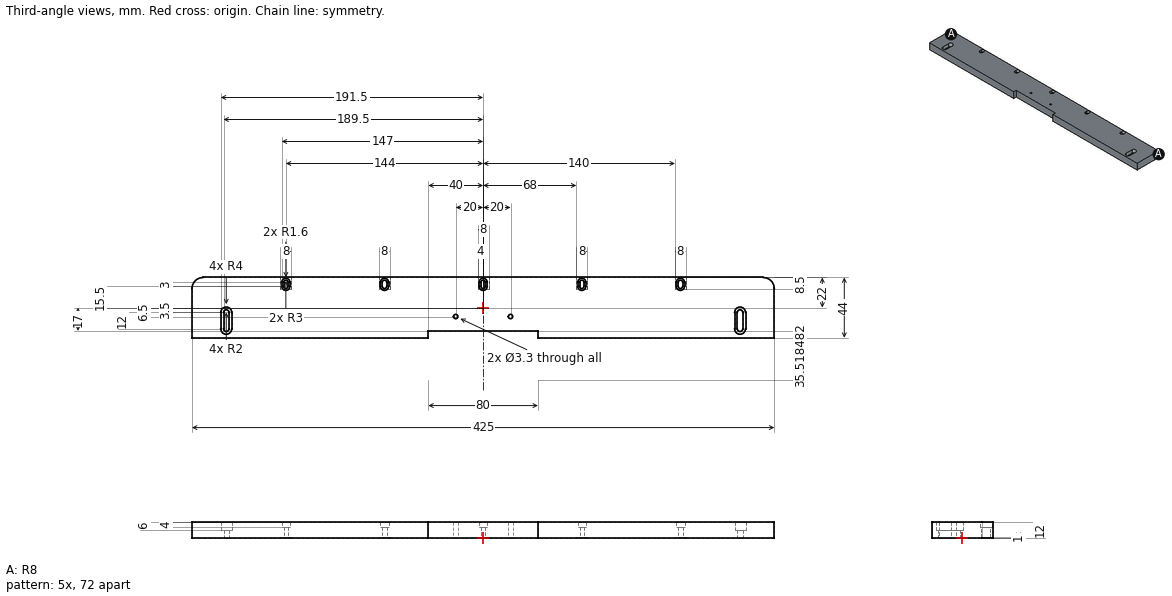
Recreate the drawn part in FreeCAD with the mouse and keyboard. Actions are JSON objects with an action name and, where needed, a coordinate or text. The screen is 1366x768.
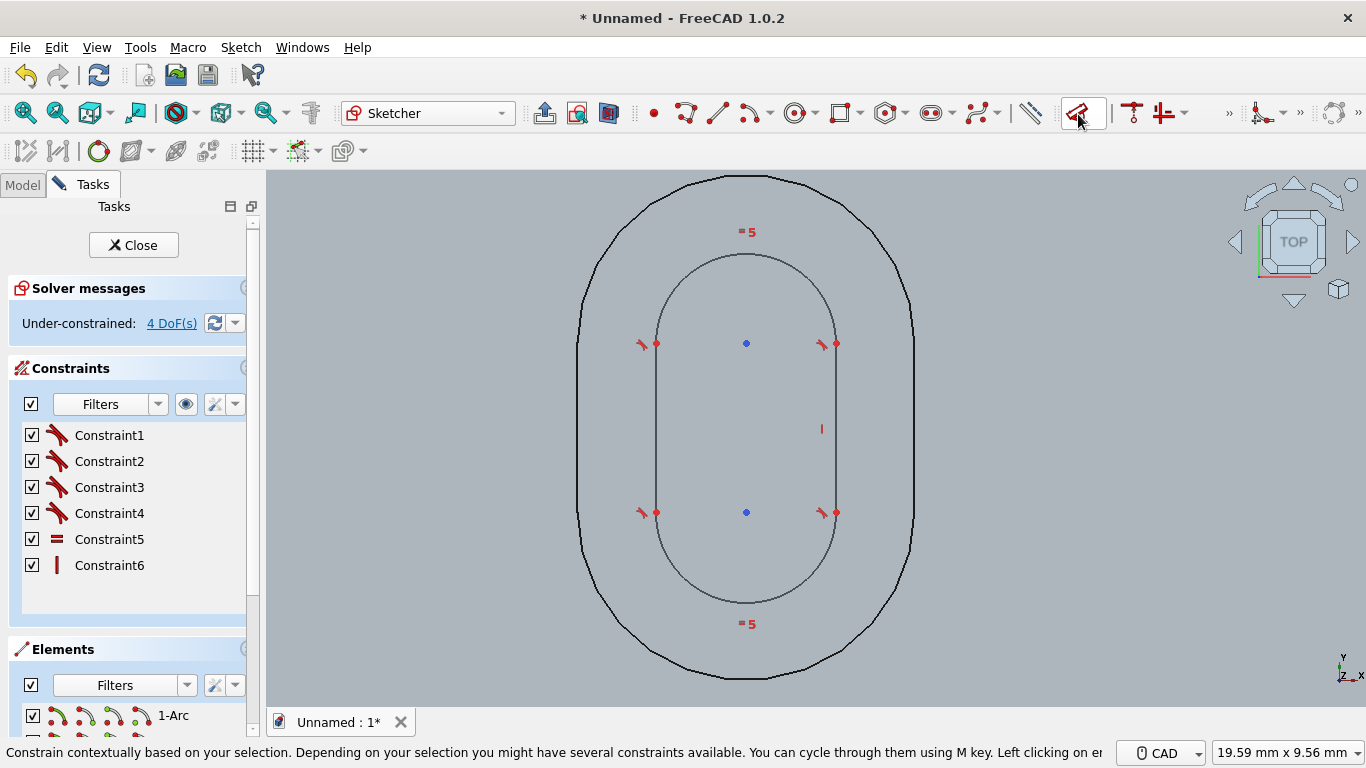
{"action": "left_click", "coordinate": [693, 586]}
{"action": "left_click", "coordinate": [674, 612]}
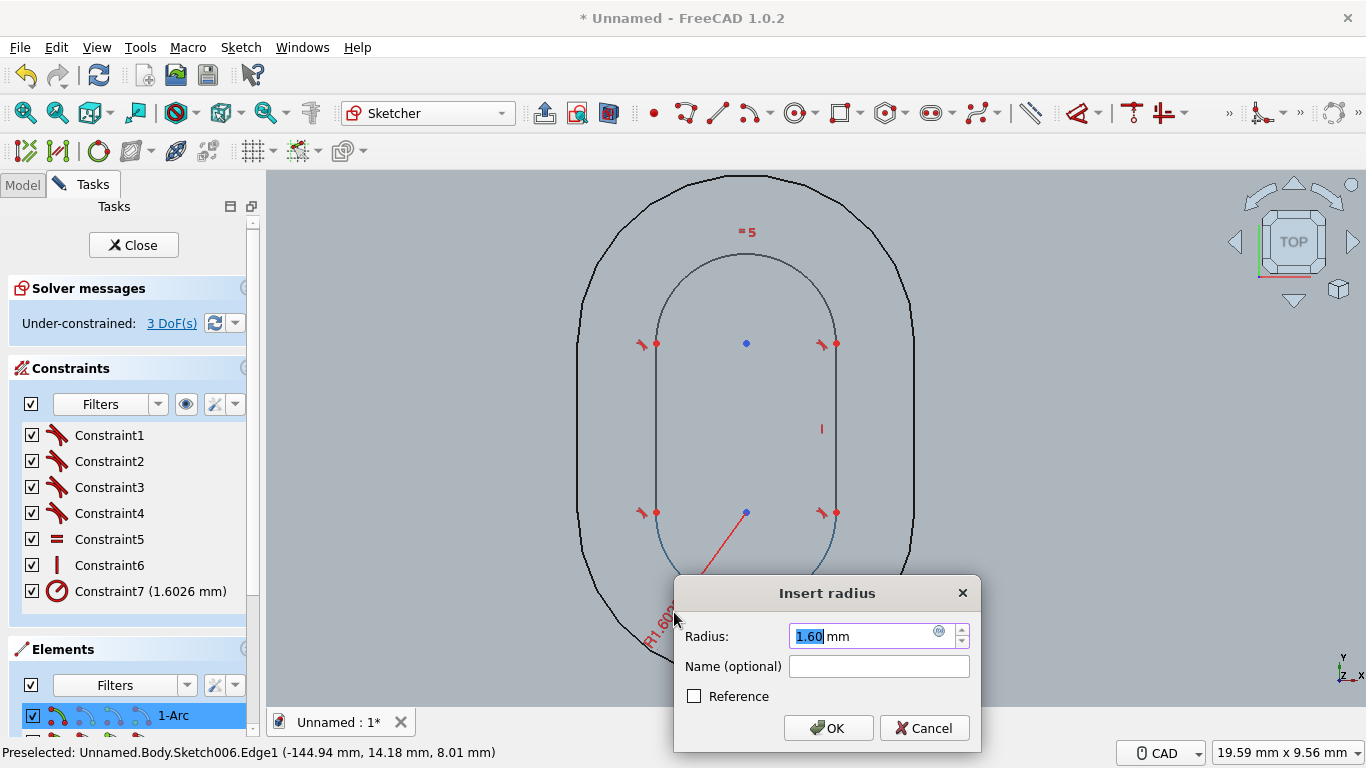
{"action": "type", "text": "1.6"}
{"action": "key", "text": "Return"}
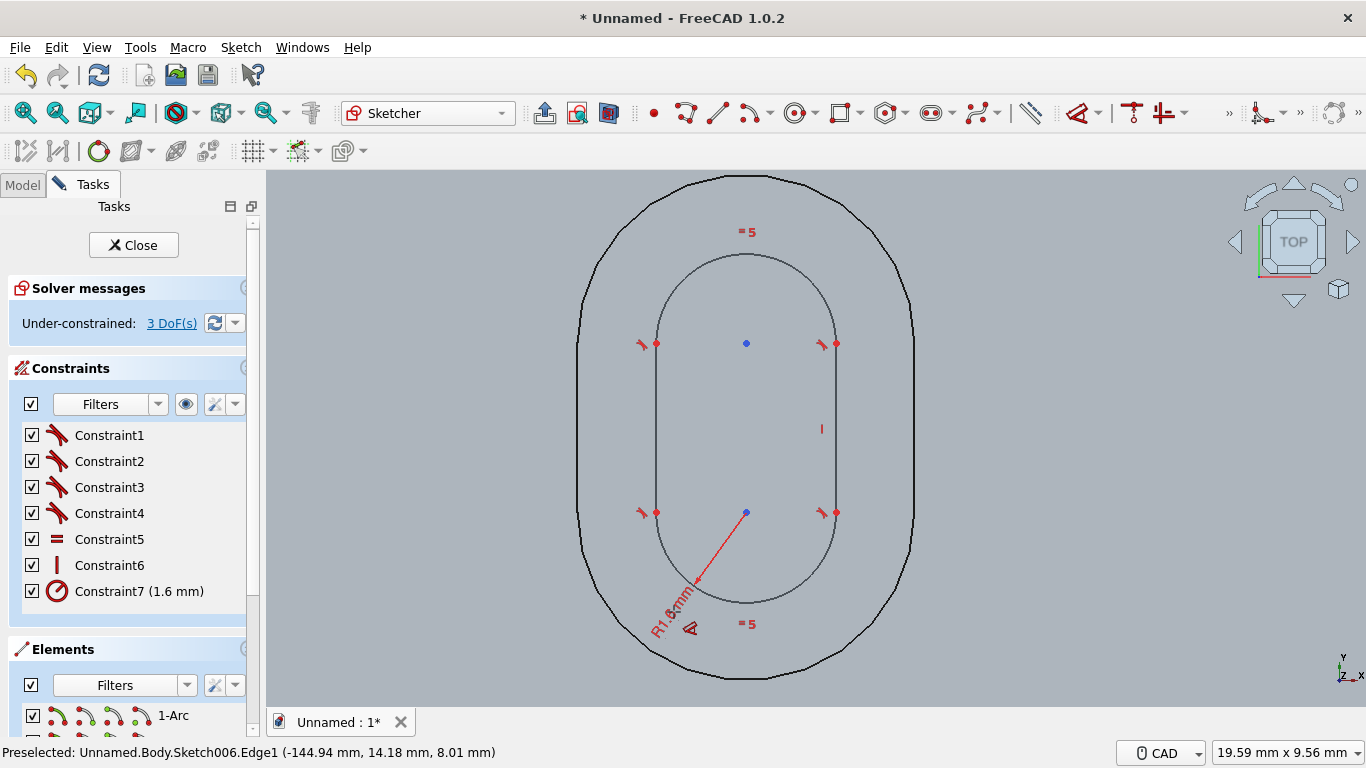
{"action": "left_click", "coordinate": [656, 462]}
{"action": "left_click", "coordinate": [622, 428]}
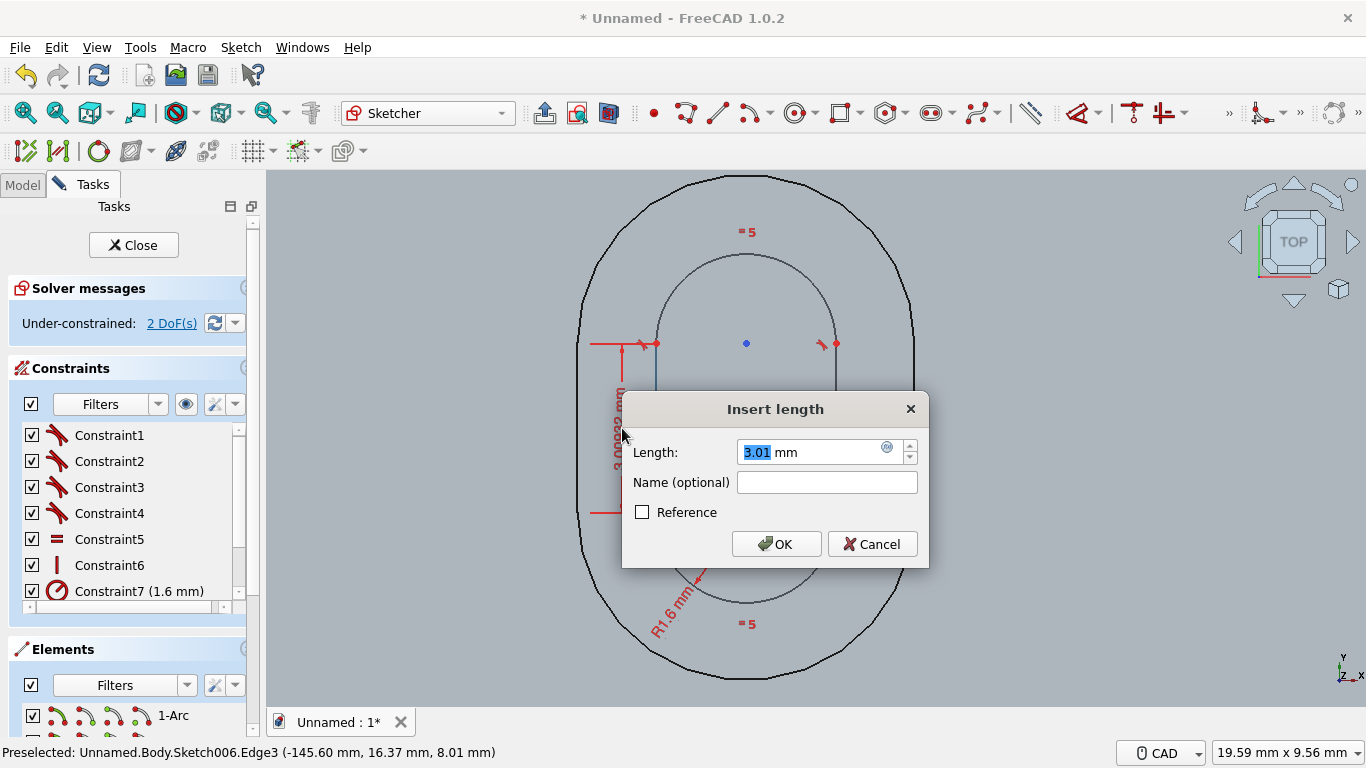
{"action": "type", "text": "3"}
{"action": "key", "text": "Return"}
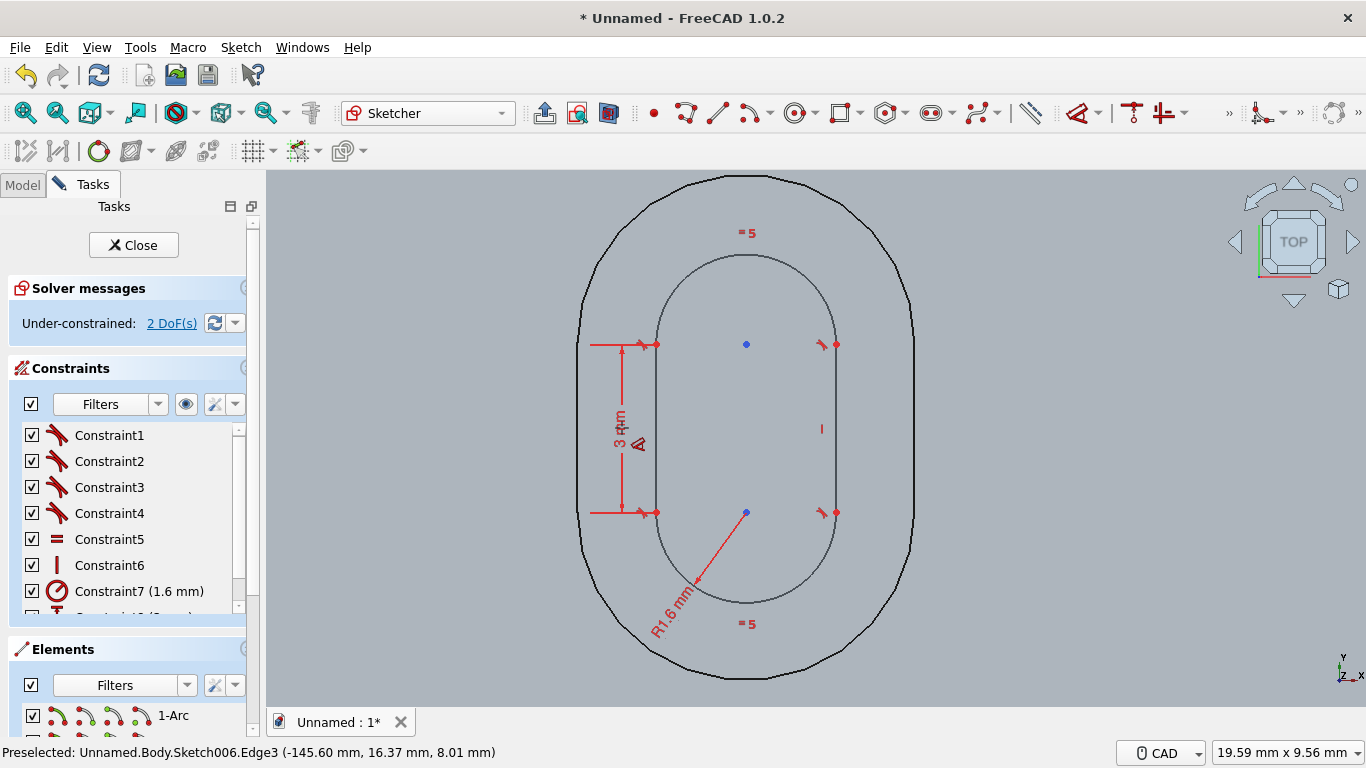
{"action": "left_click", "coordinate": [746, 513]}
{"action": "left_click", "coordinate": [974, 479]}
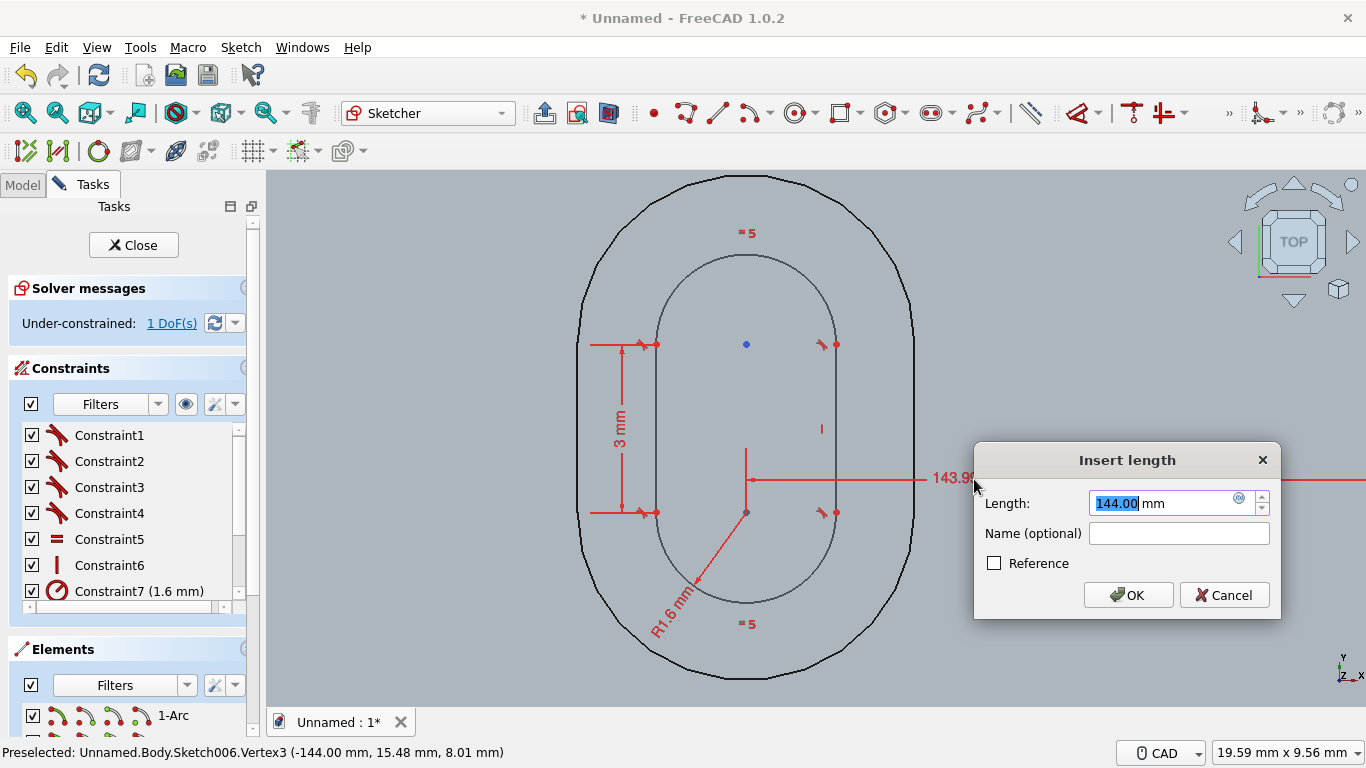
{"action": "type", "text": "144"}
{"action": "key", "text": "Return"}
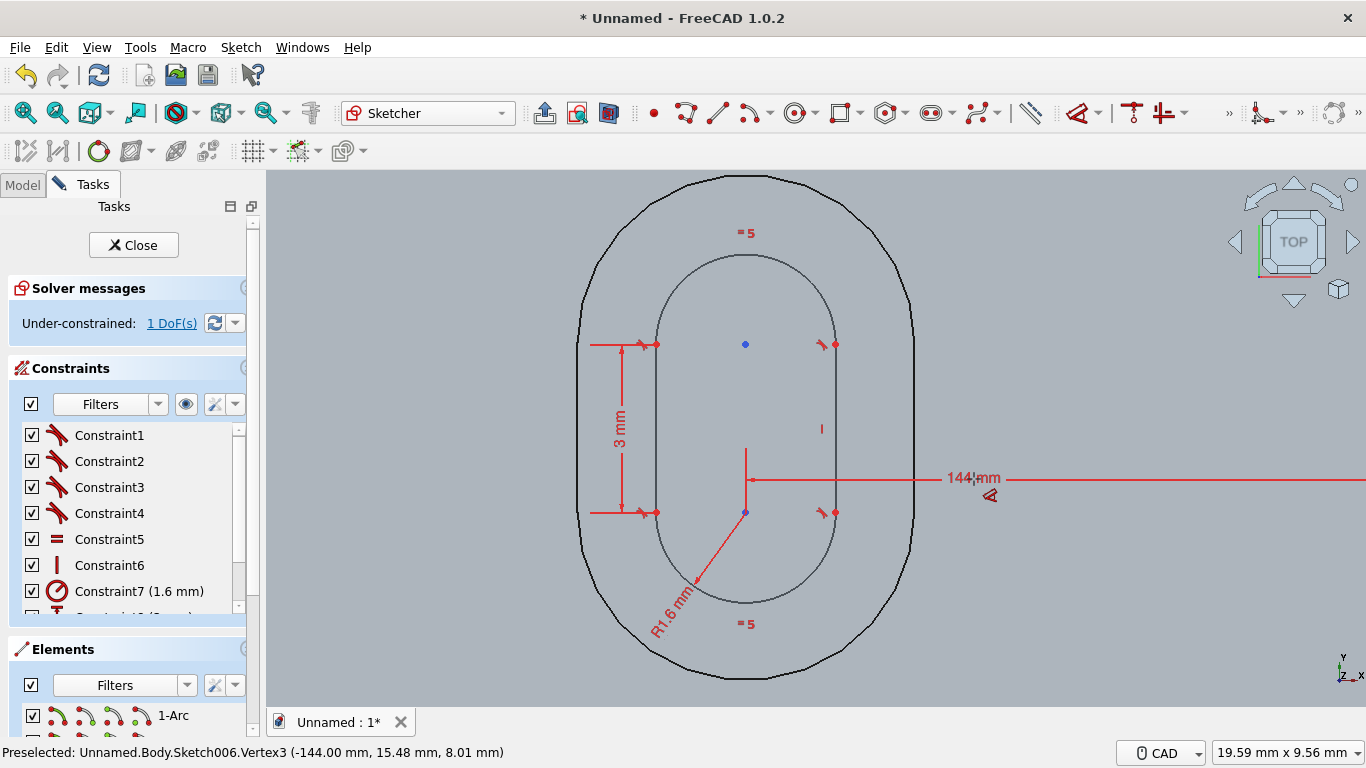
{"action": "left_click", "coordinate": [656, 513]}
{"action": "left_click", "coordinate": [622, 558]}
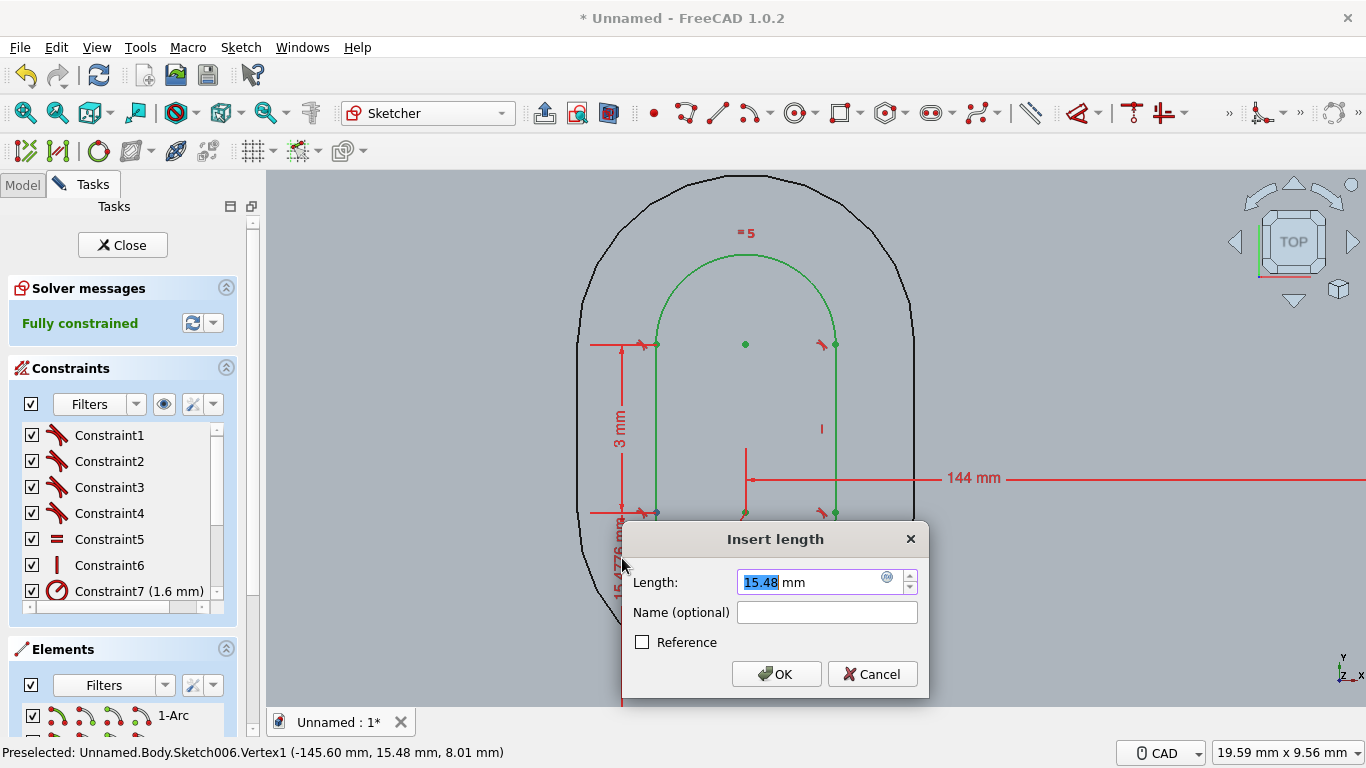
{"action": "type", "text": "15.5"}
{"action": "key", "text": "Return"}
{"action": "key", "text": "Escape"}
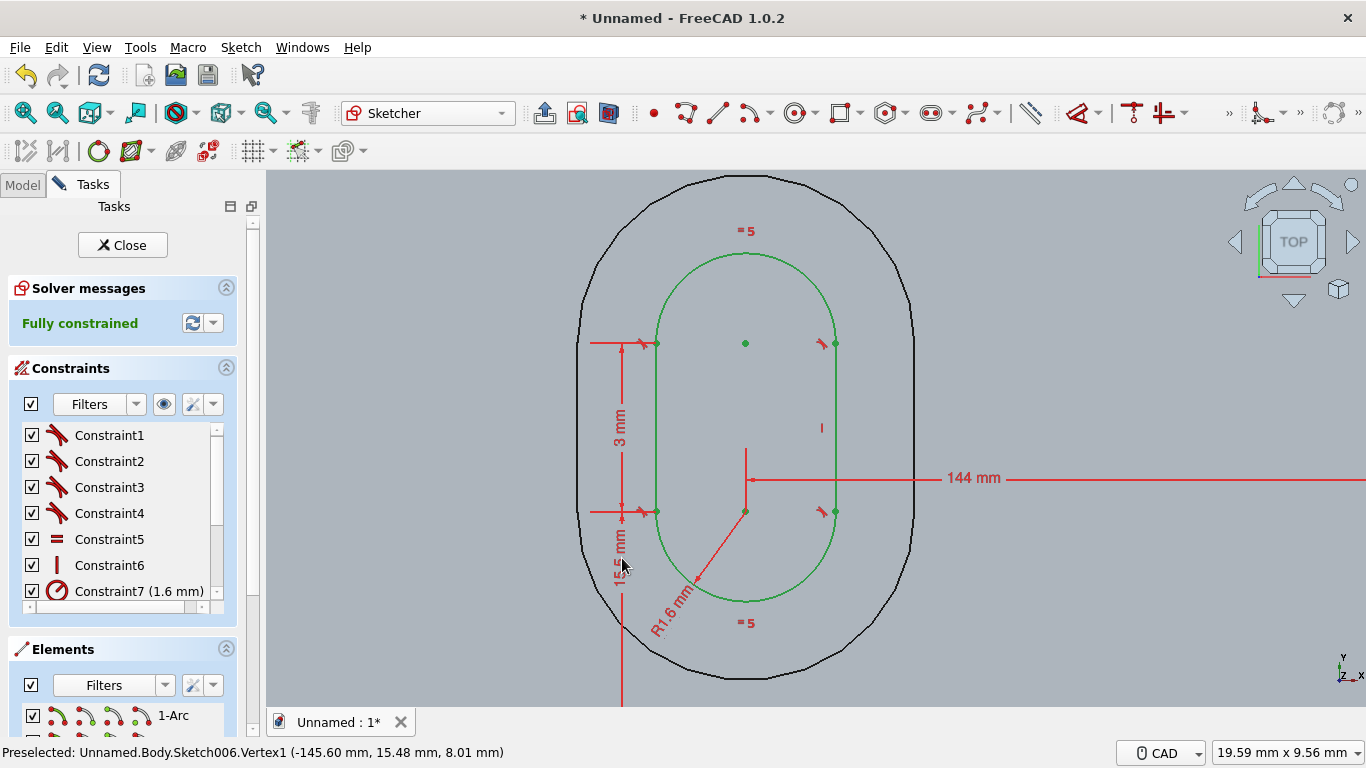
{"action": "left_click", "coordinate": [123, 245]}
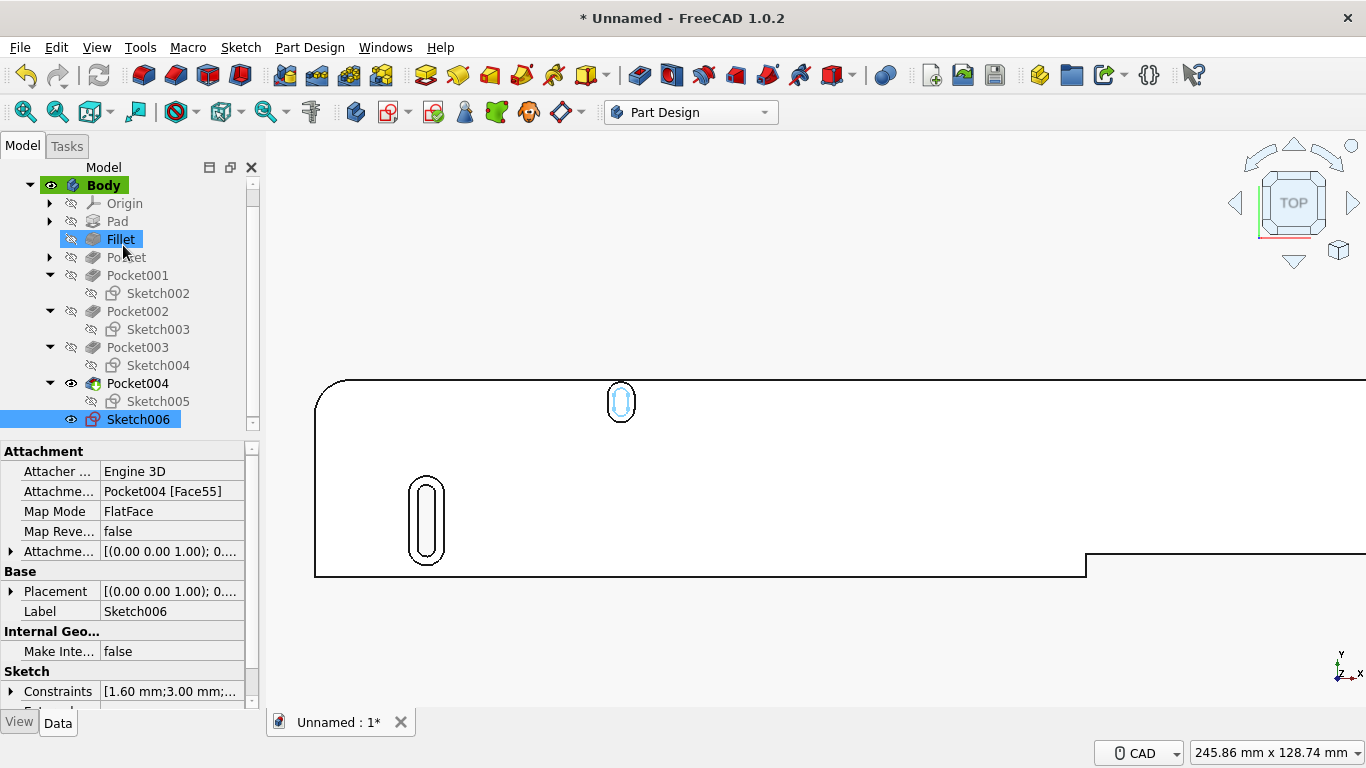
{"action": "left_click", "coordinate": [640, 76]}